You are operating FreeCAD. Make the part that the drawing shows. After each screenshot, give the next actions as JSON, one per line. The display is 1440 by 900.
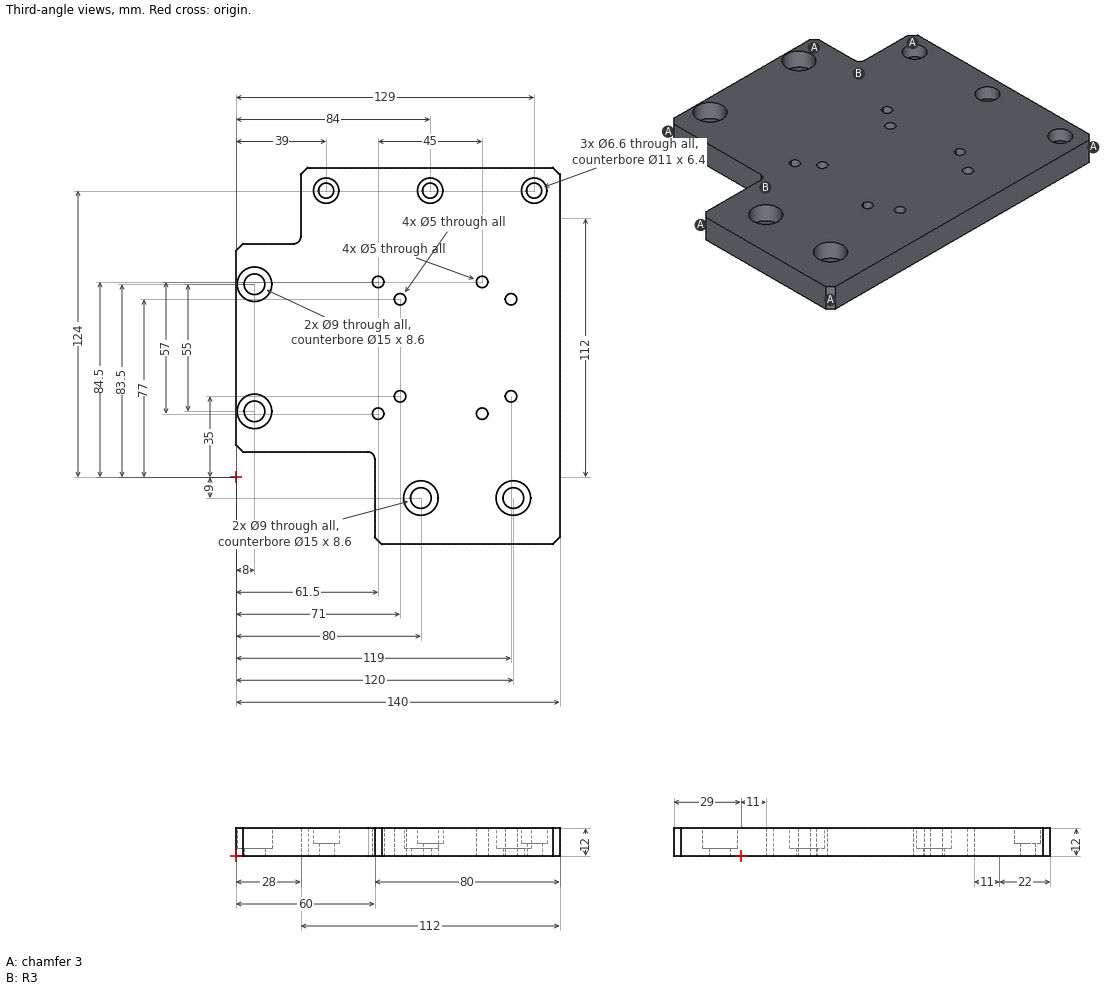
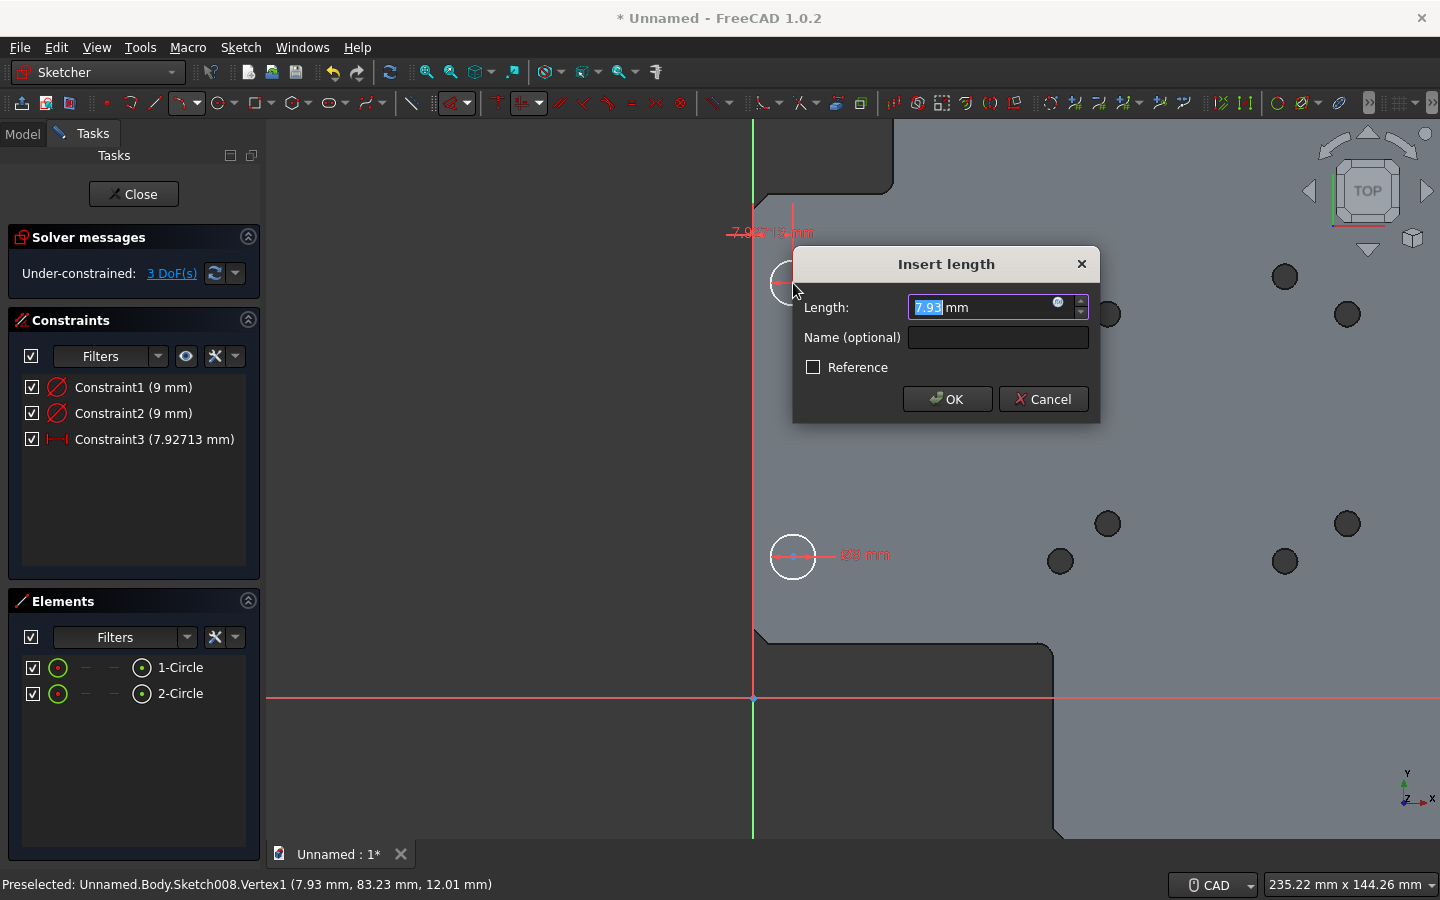
{"action": "type", "text": "8"}
{"action": "key", "text": "Return"}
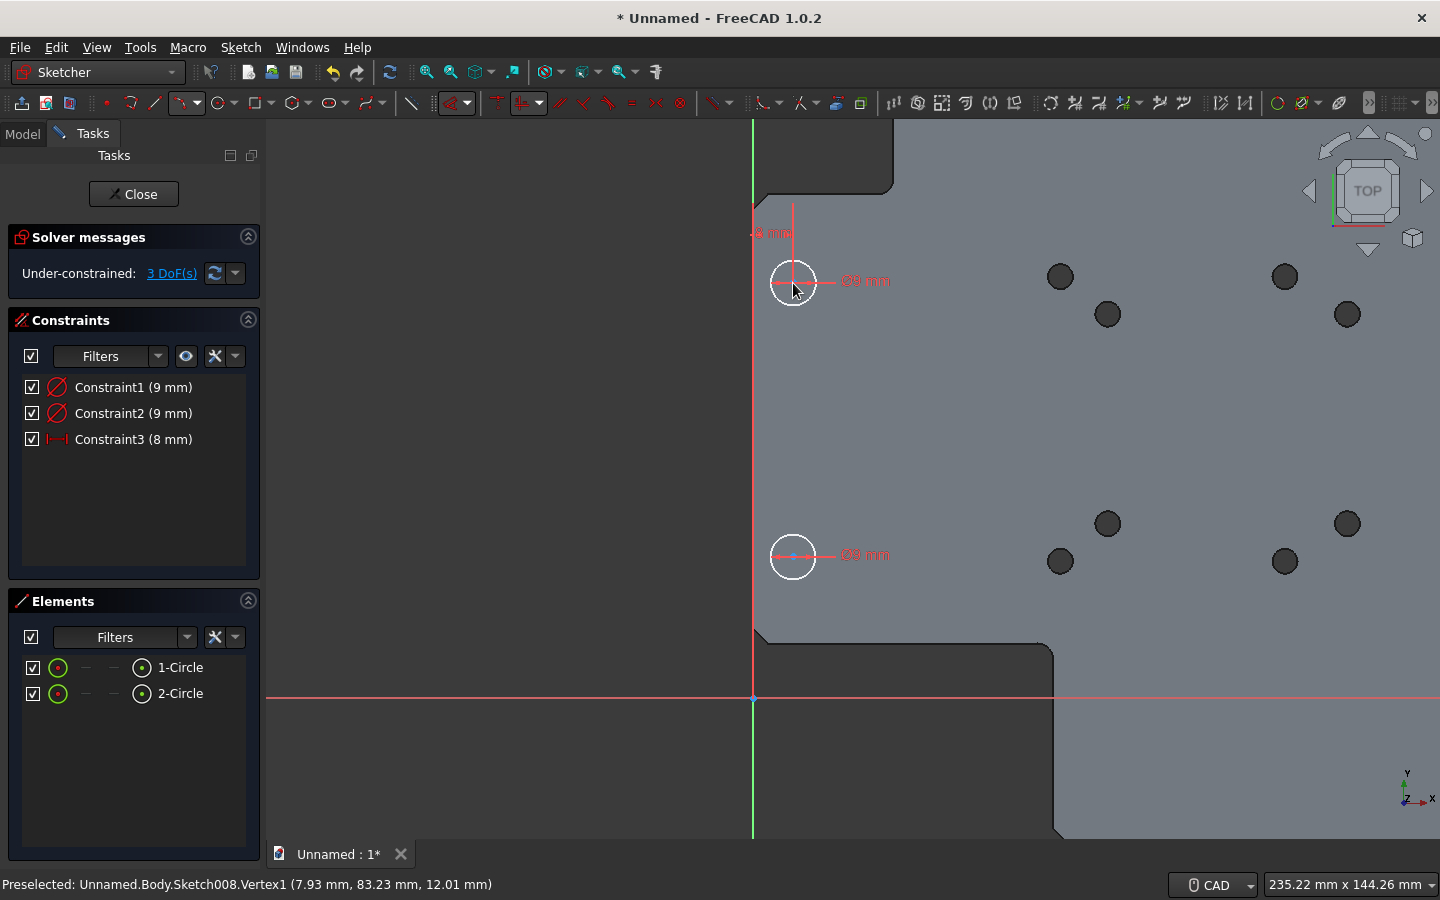
{"action": "left_click", "coordinate": [793, 557]}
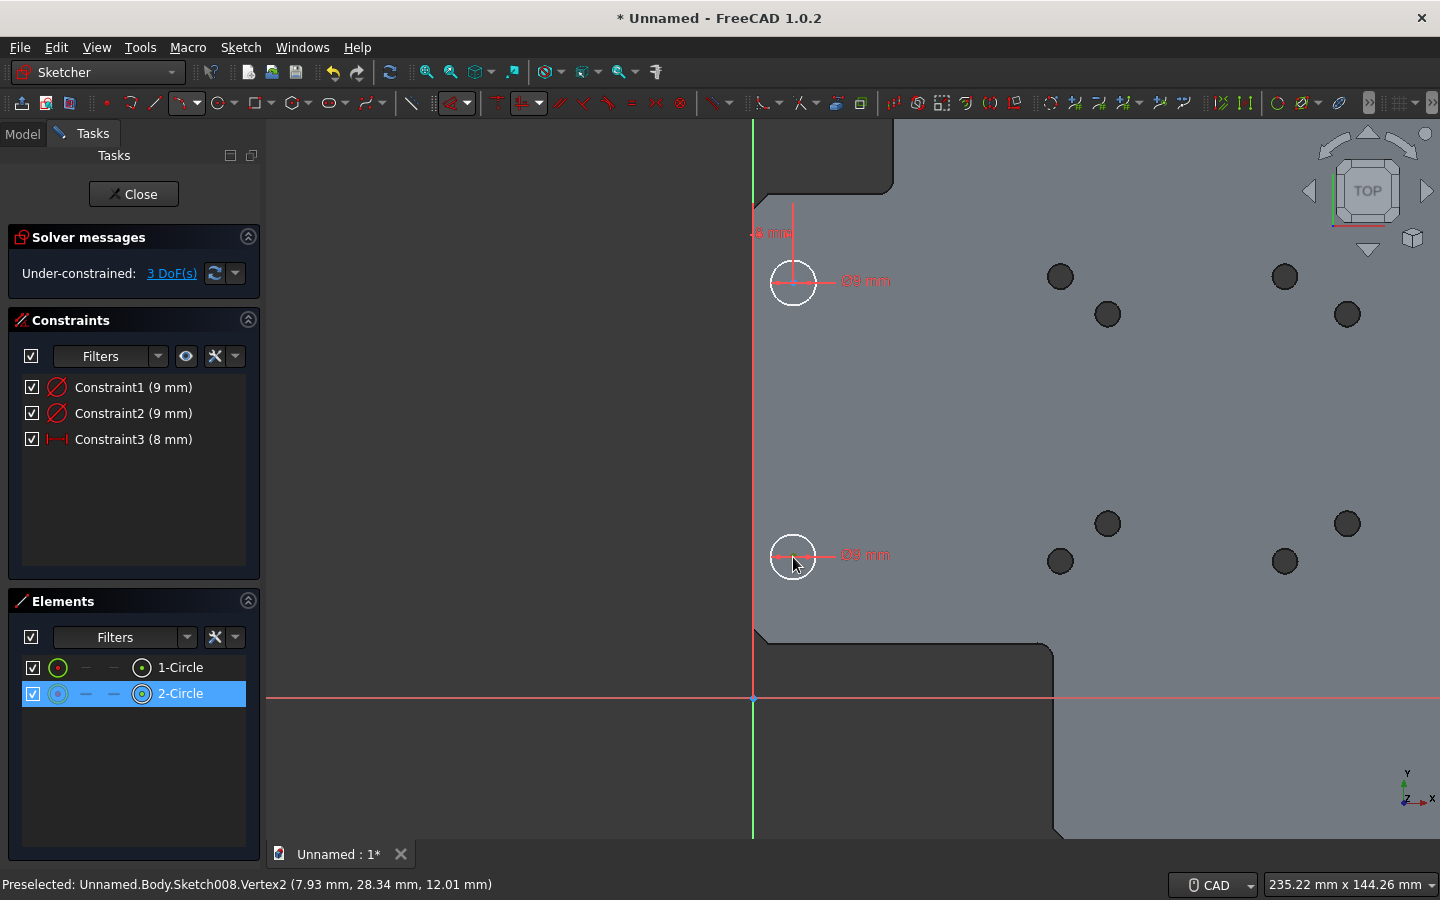
{"action": "left_click", "coordinate": [470, 104]}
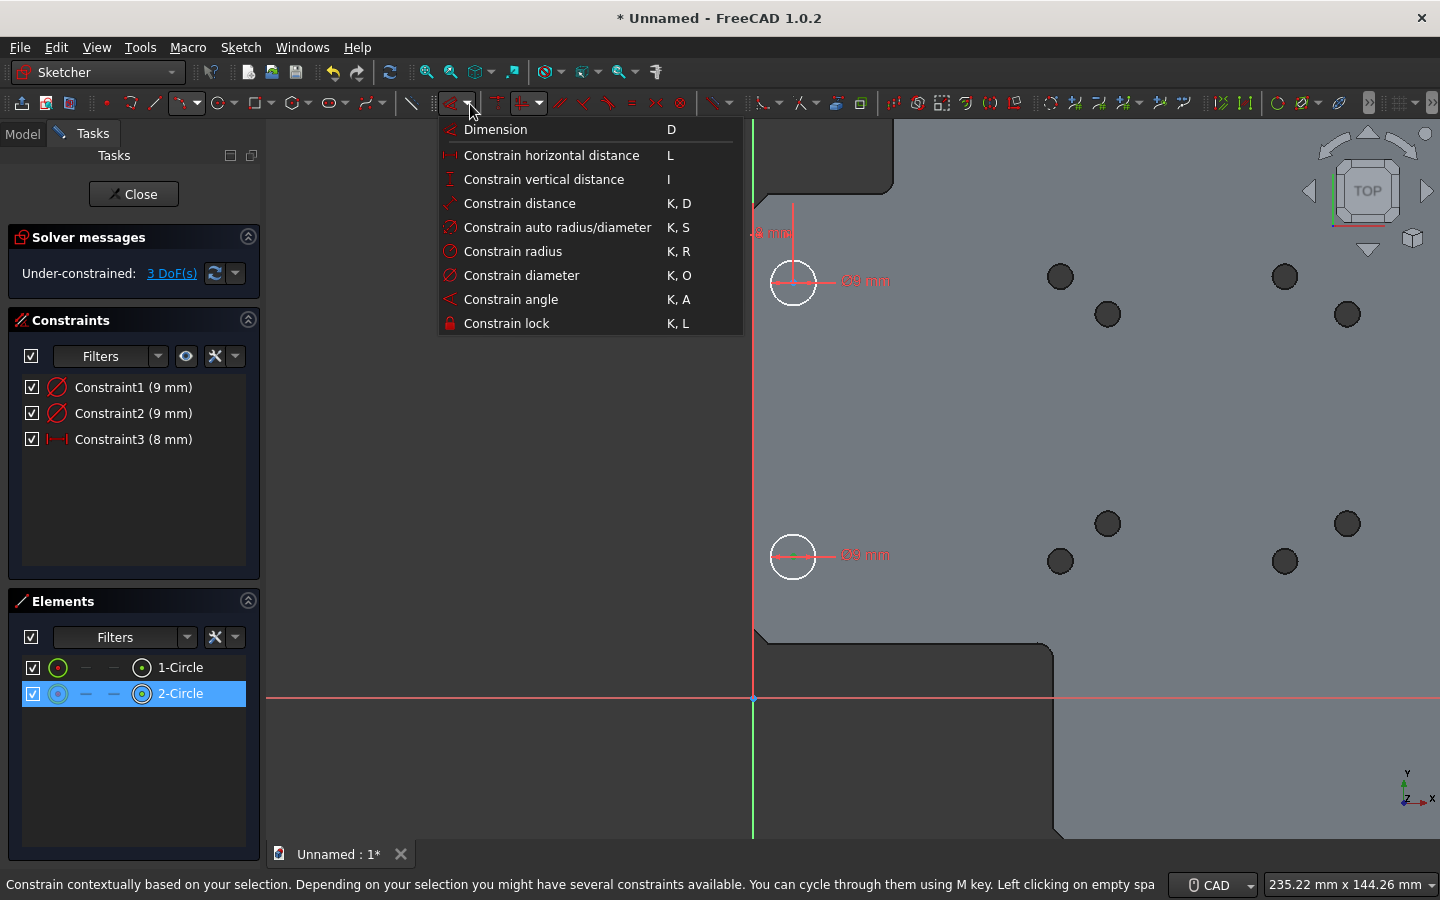
{"action": "left_click", "coordinate": [591, 155]}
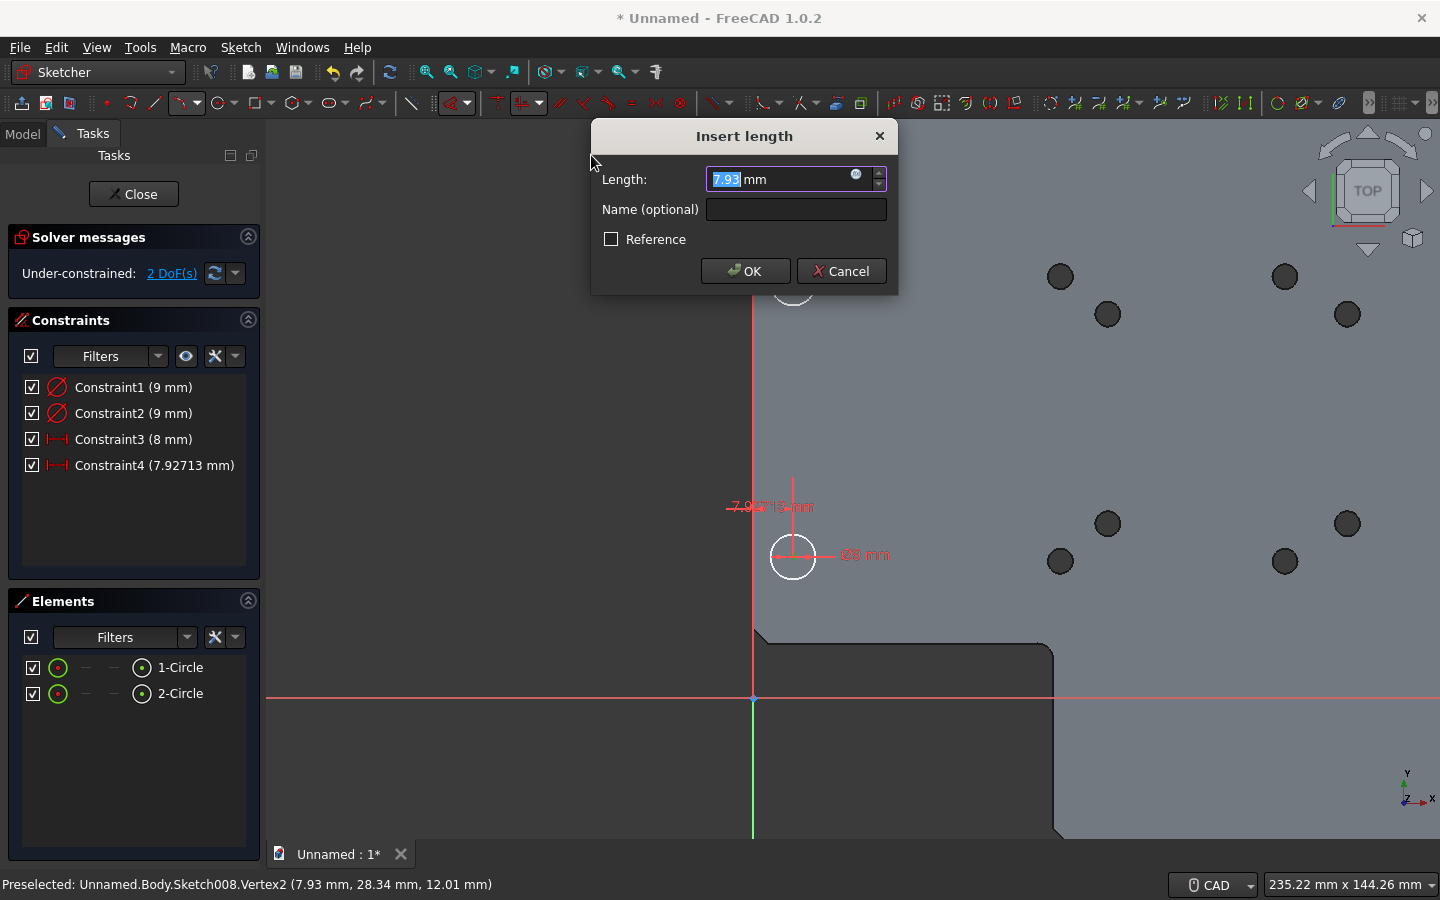
{"action": "type", "text": "8"}
{"action": "key", "text": "Return"}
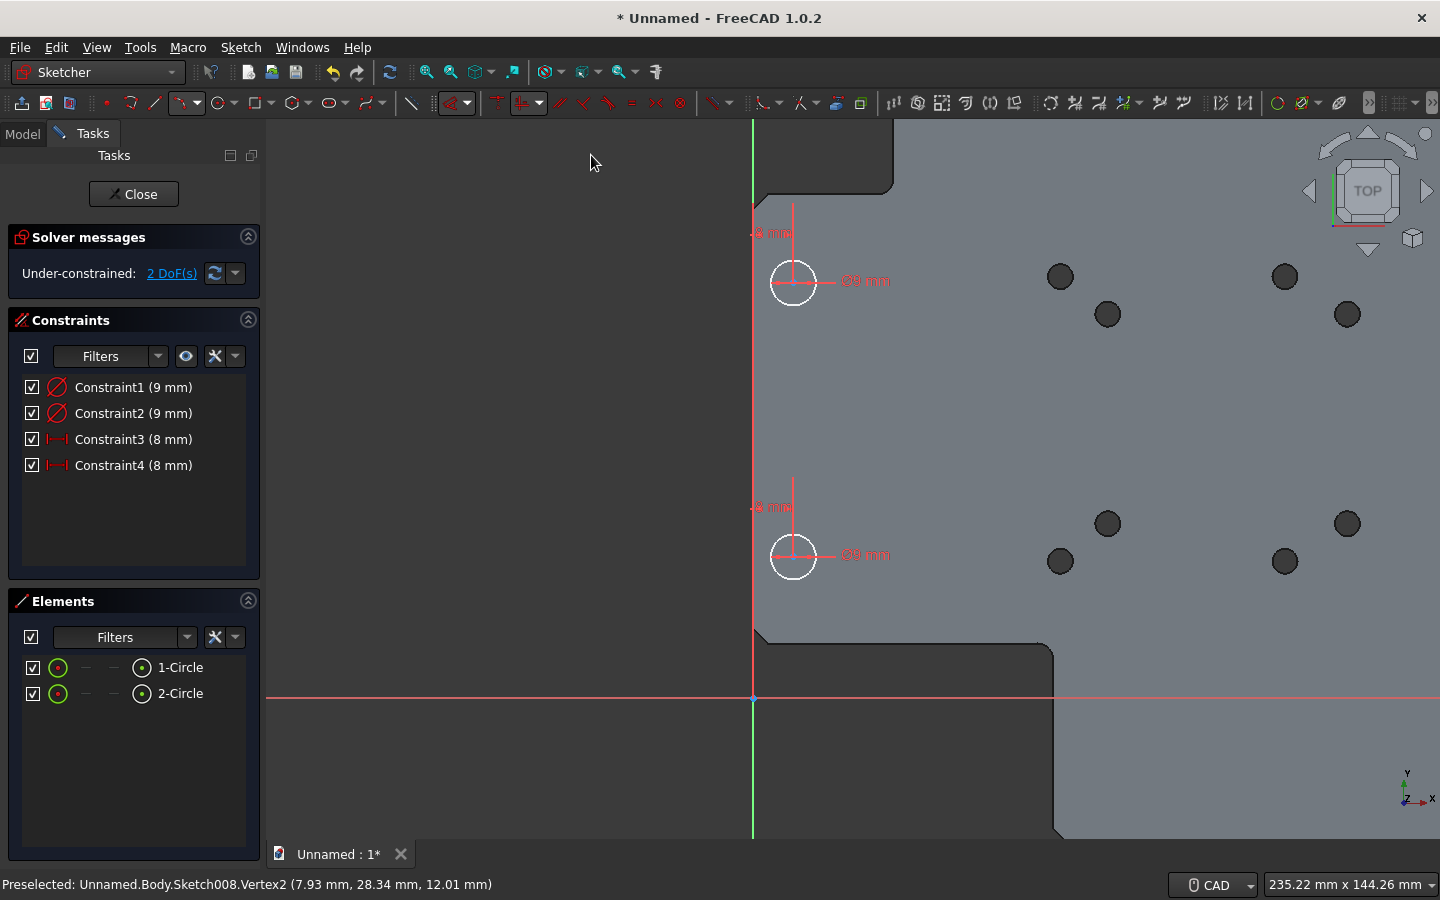
{"action": "left_click", "coordinate": [793, 283]}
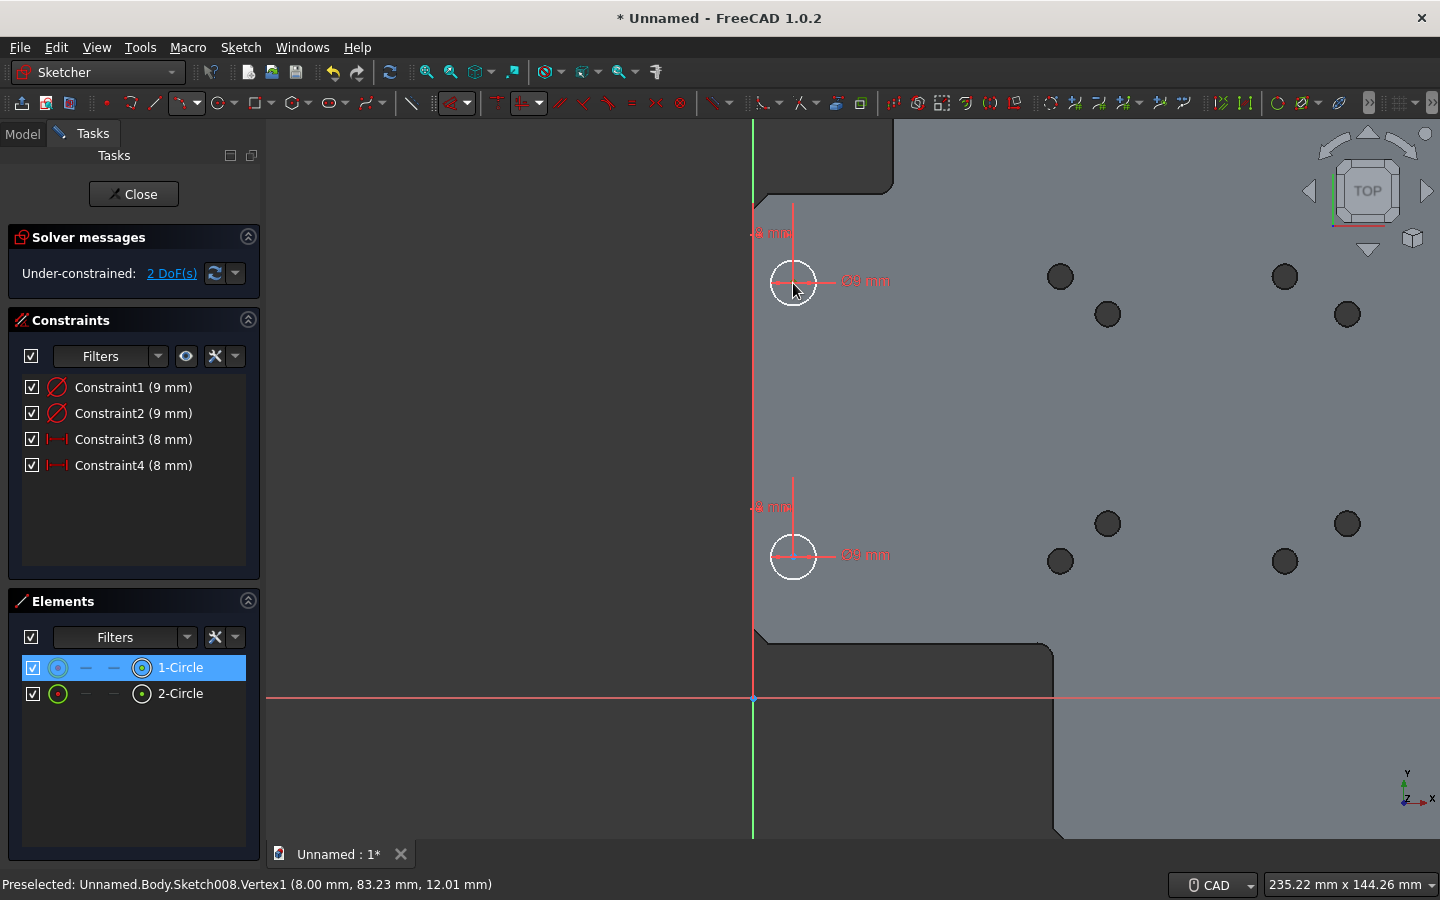
{"action": "left_click", "coordinate": [793, 557]}